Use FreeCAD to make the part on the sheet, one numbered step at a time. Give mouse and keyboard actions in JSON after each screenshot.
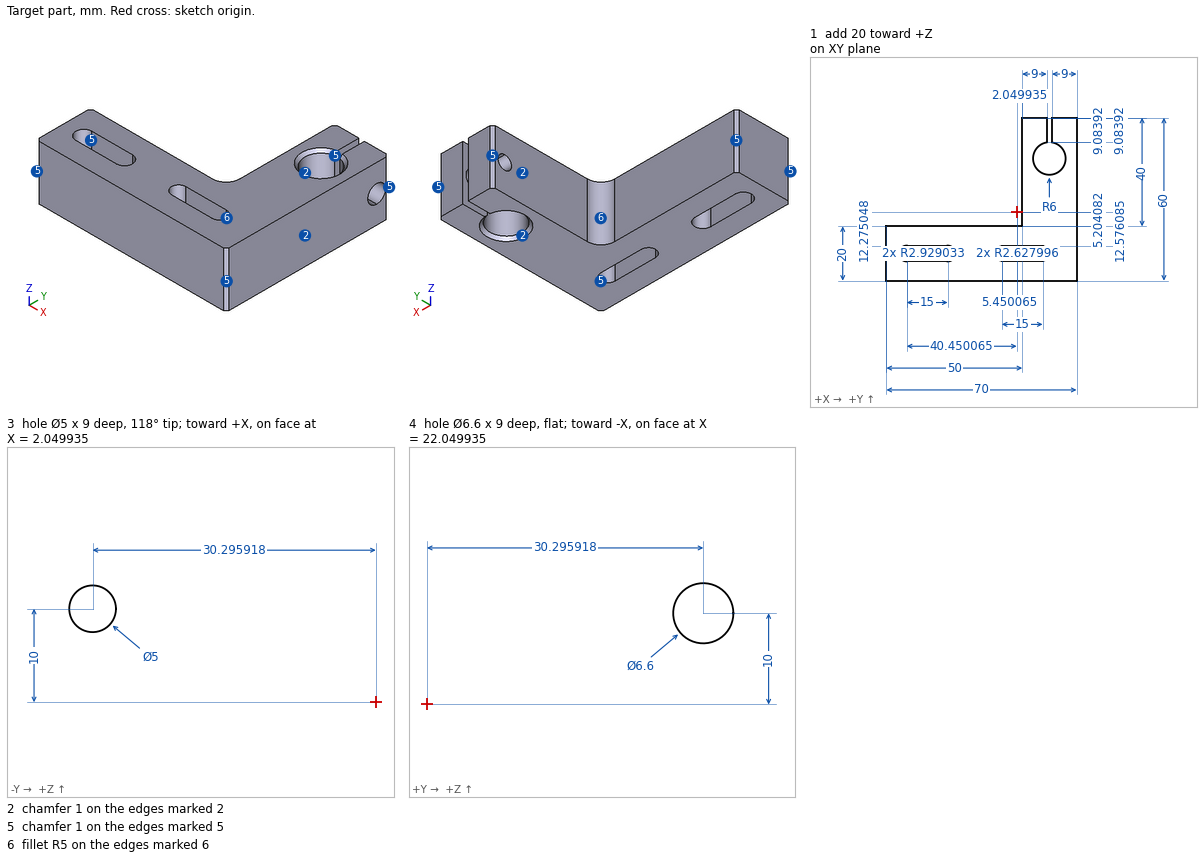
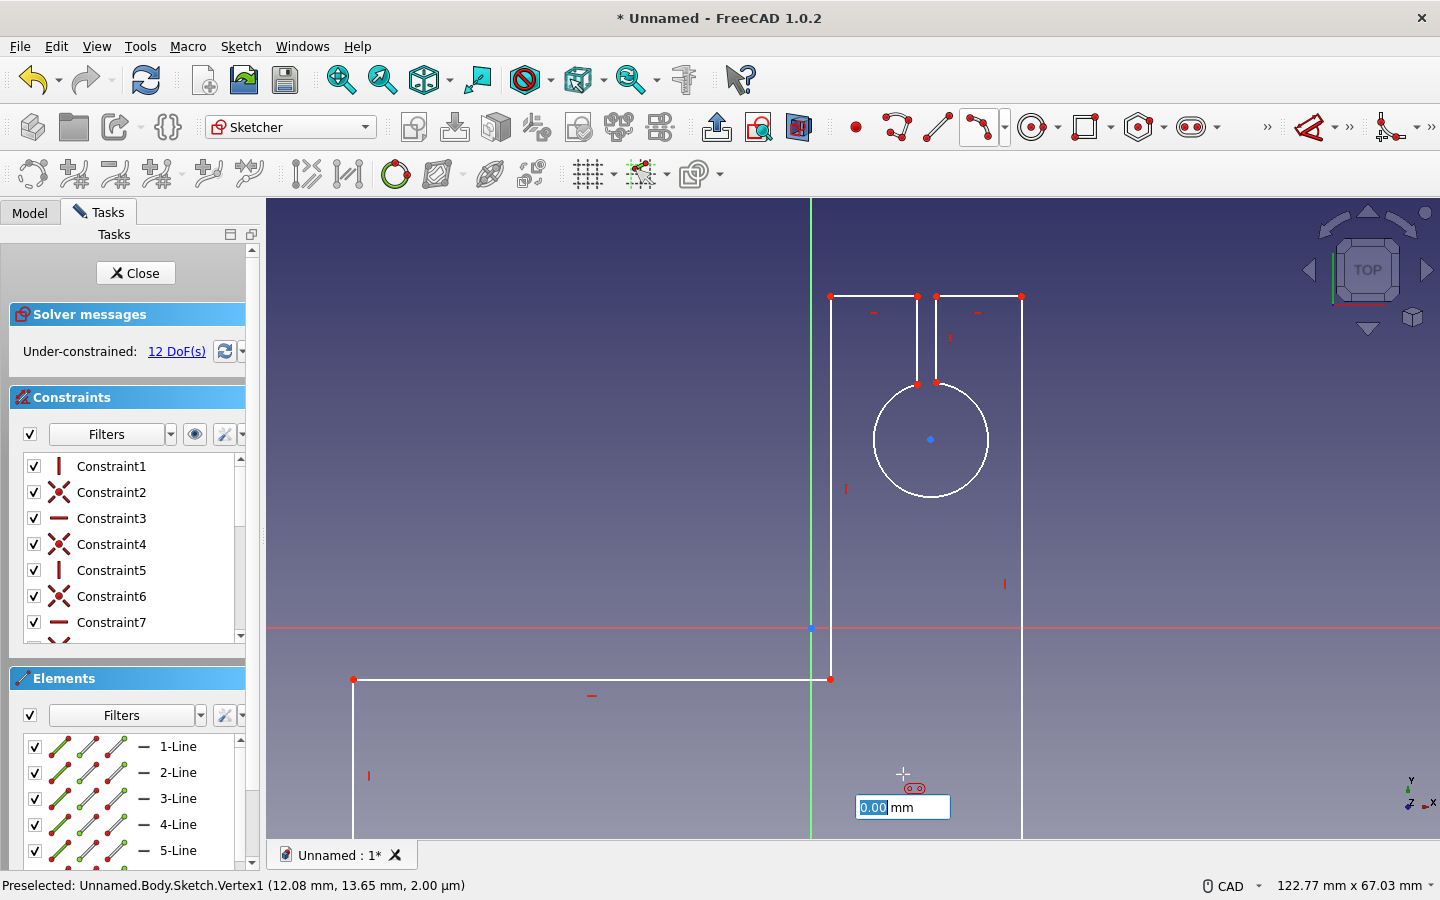
{"action": "left_click", "coordinate": [831, 749]}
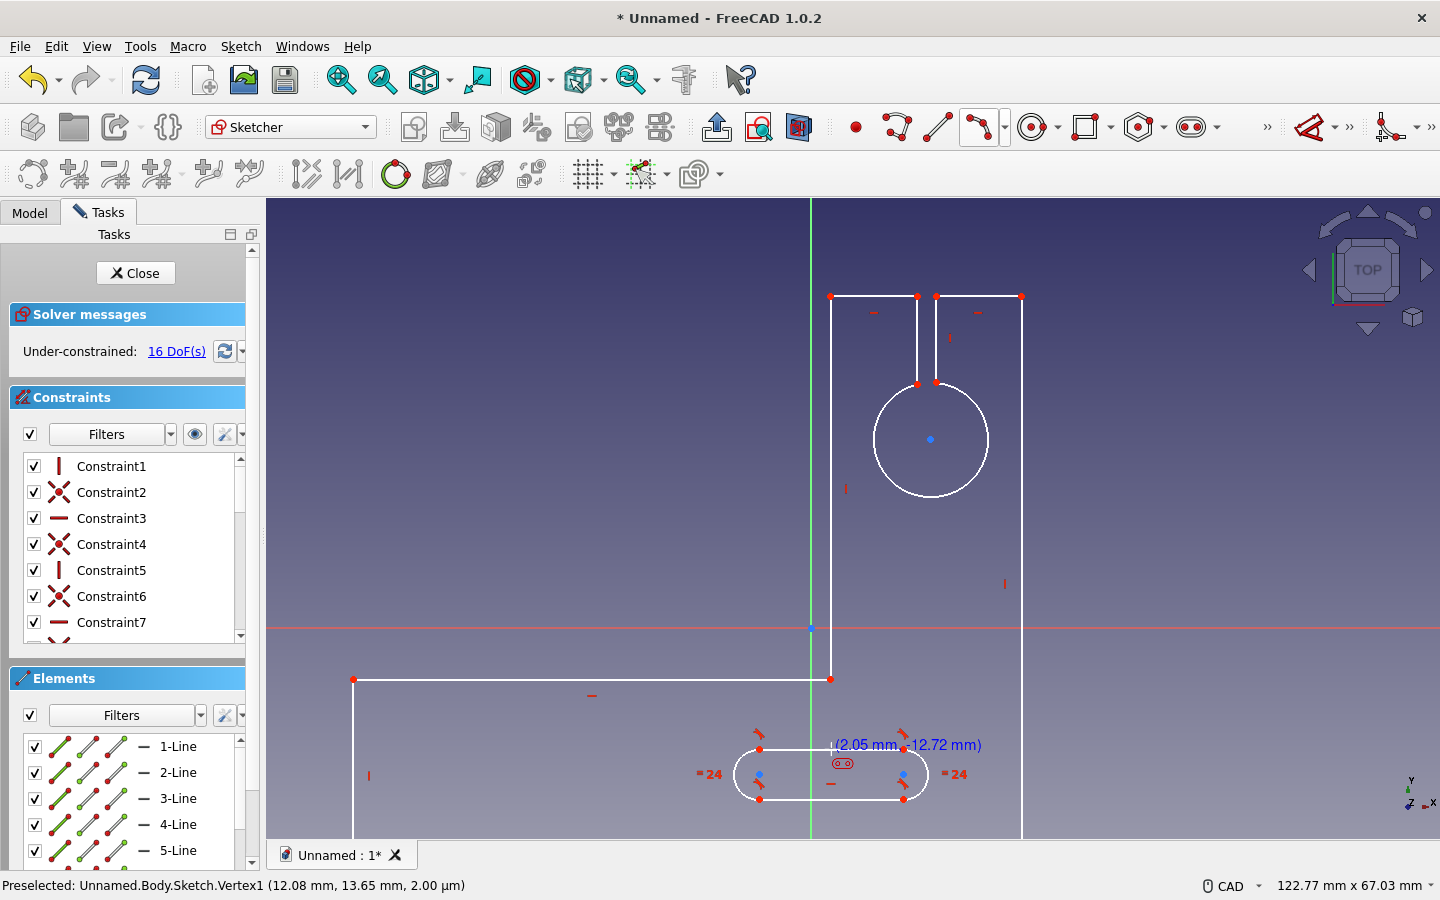
{"action": "left_click", "coordinate": [425, 774]}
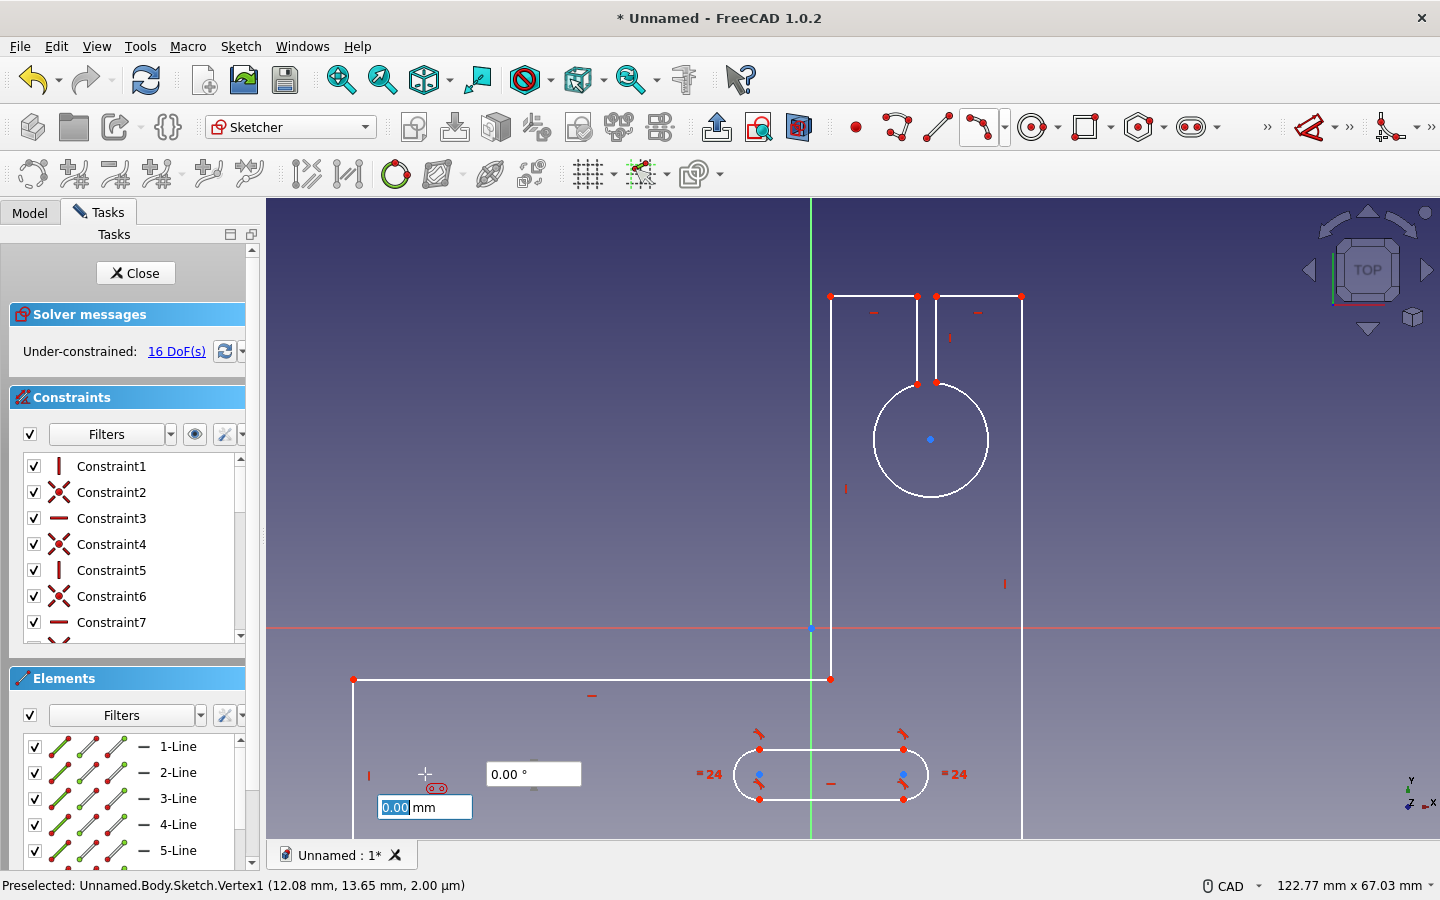
{"action": "left_click", "coordinate": [568, 774]}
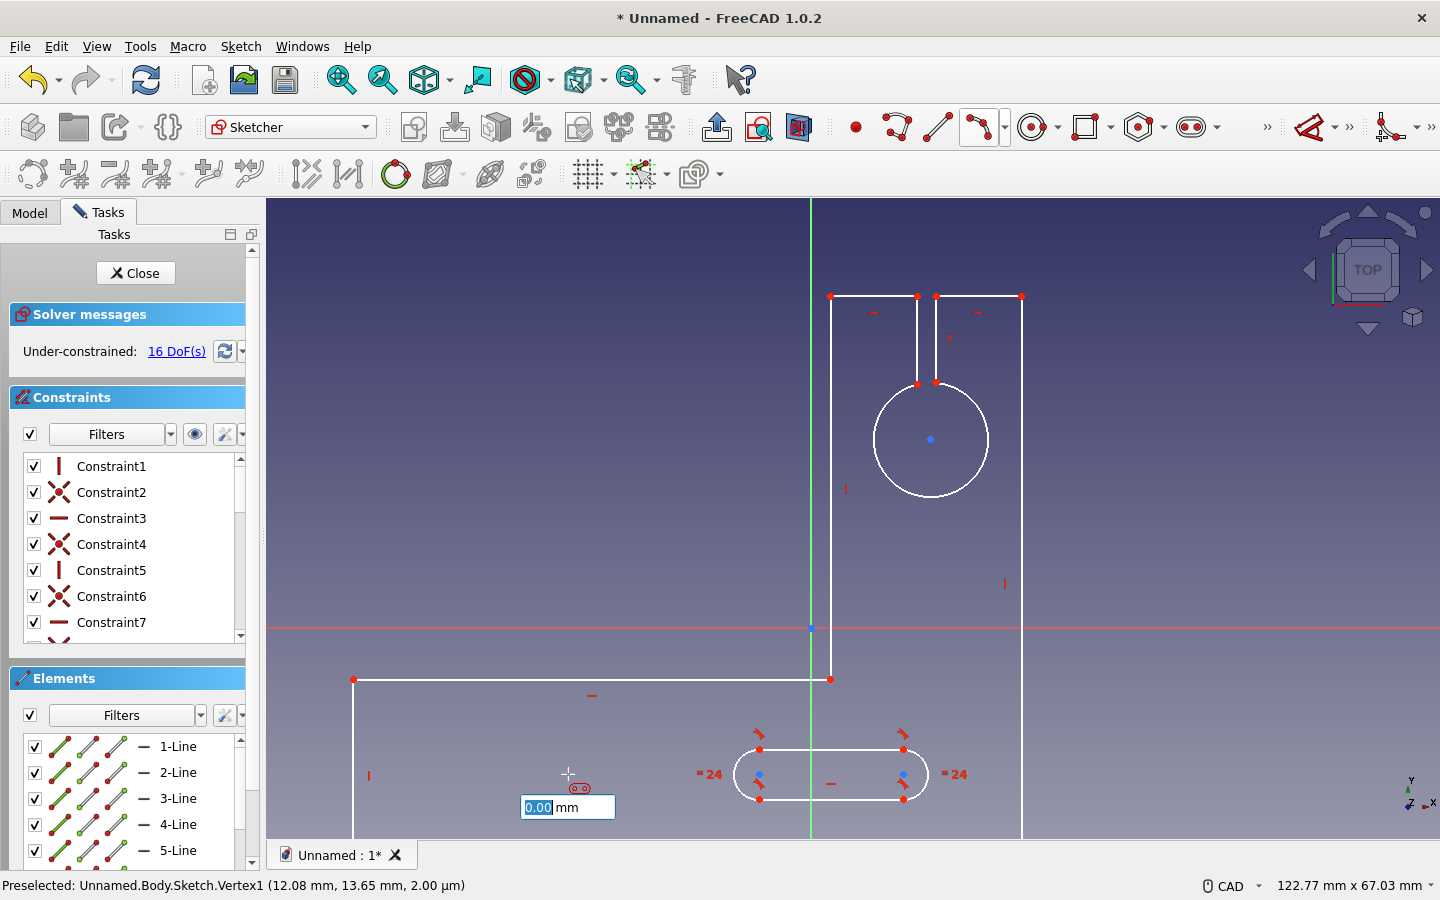
{"action": "left_click", "coordinate": [496, 746]}
{"action": "key", "text": "Escape"}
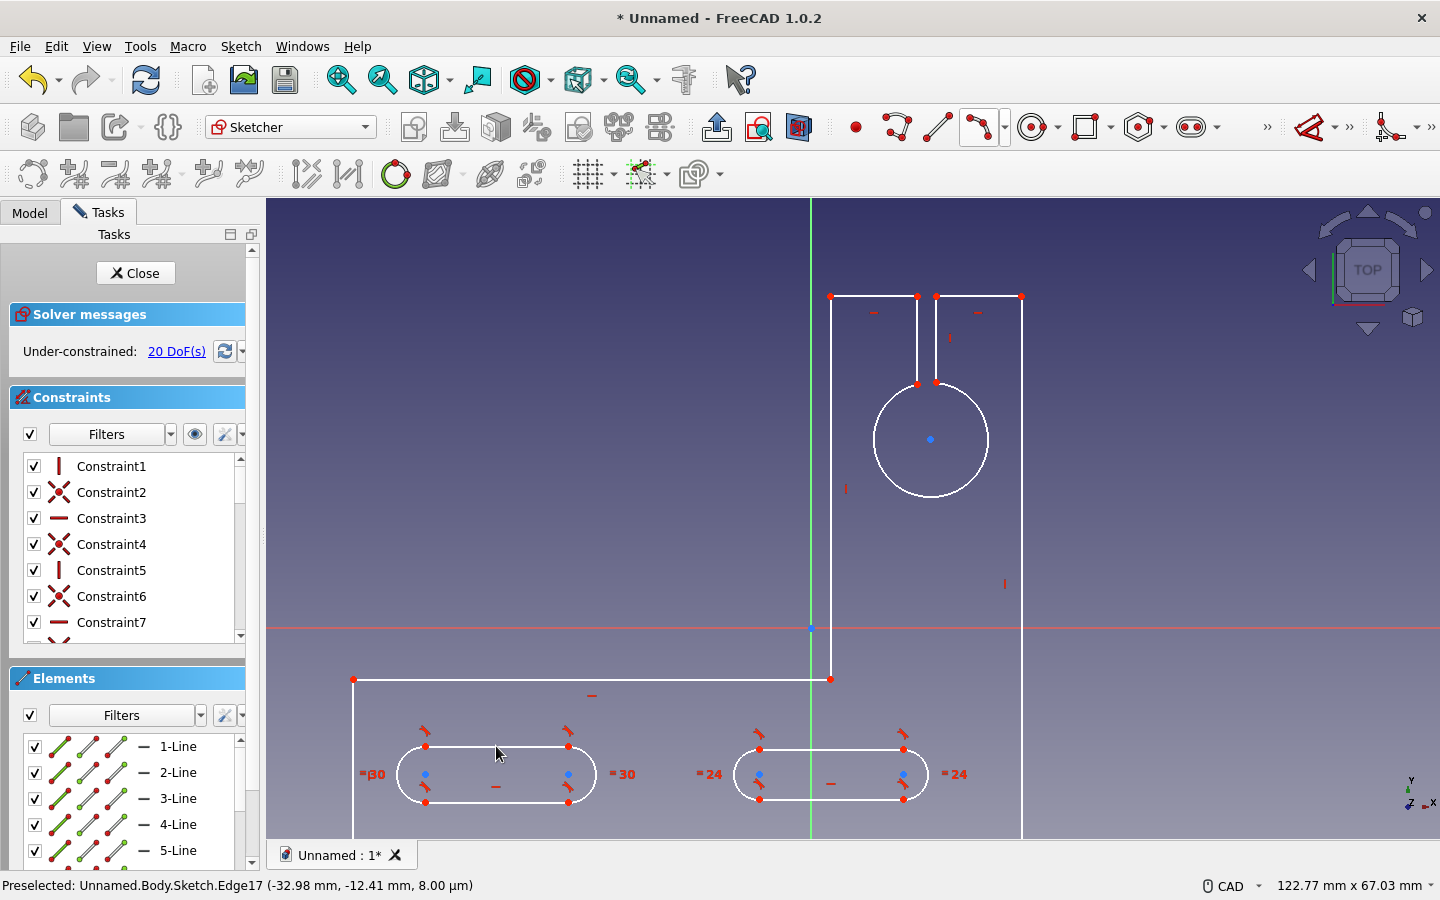
{"action": "left_click", "coordinate": [1308, 128]}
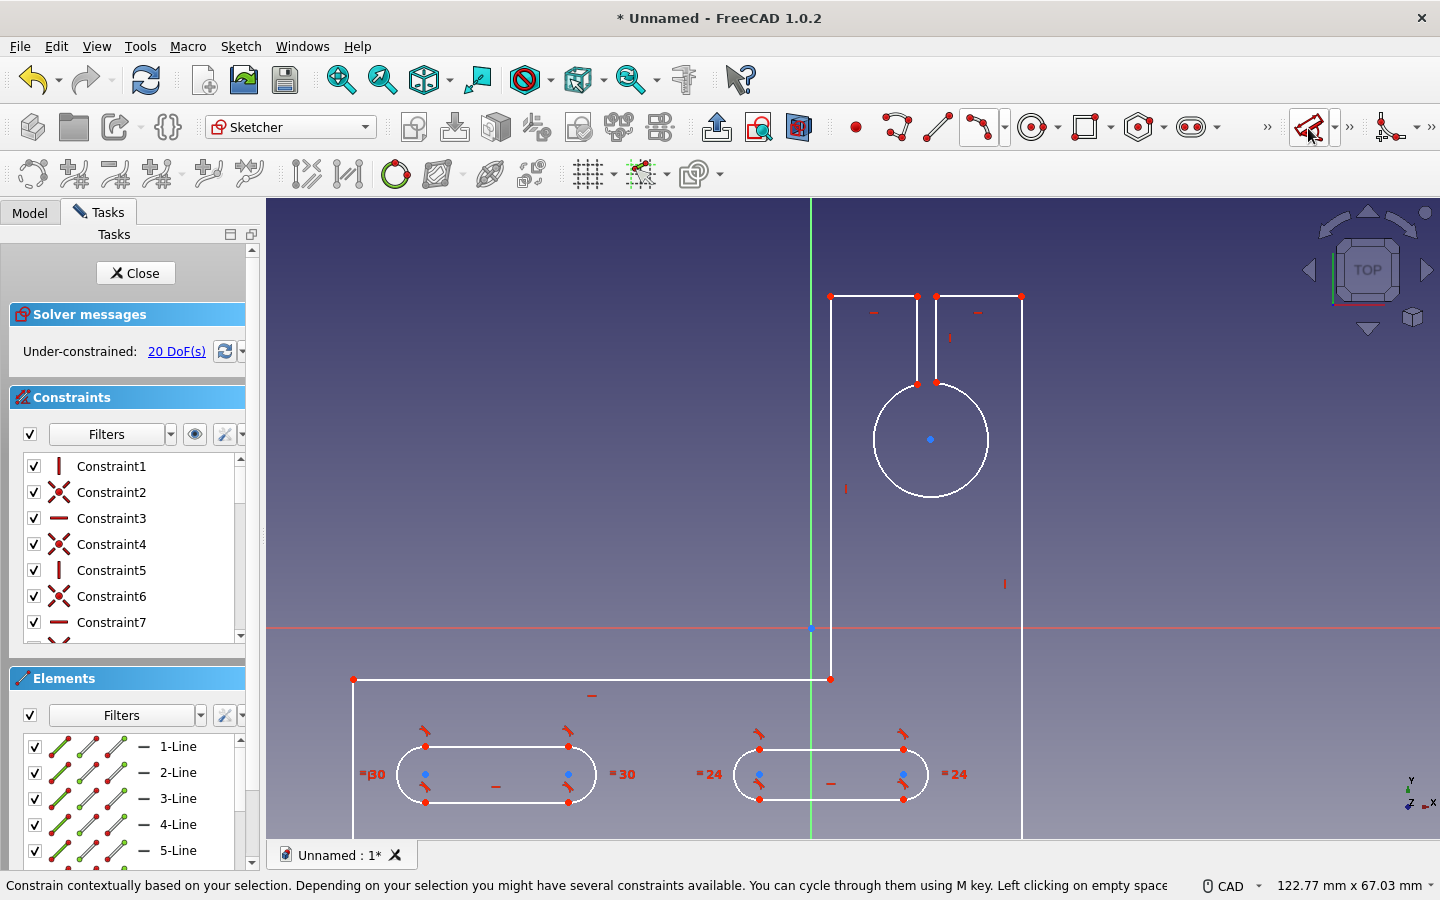
{"action": "left_click", "coordinate": [880, 465]}
{"action": "left_click", "coordinate": [851, 479]}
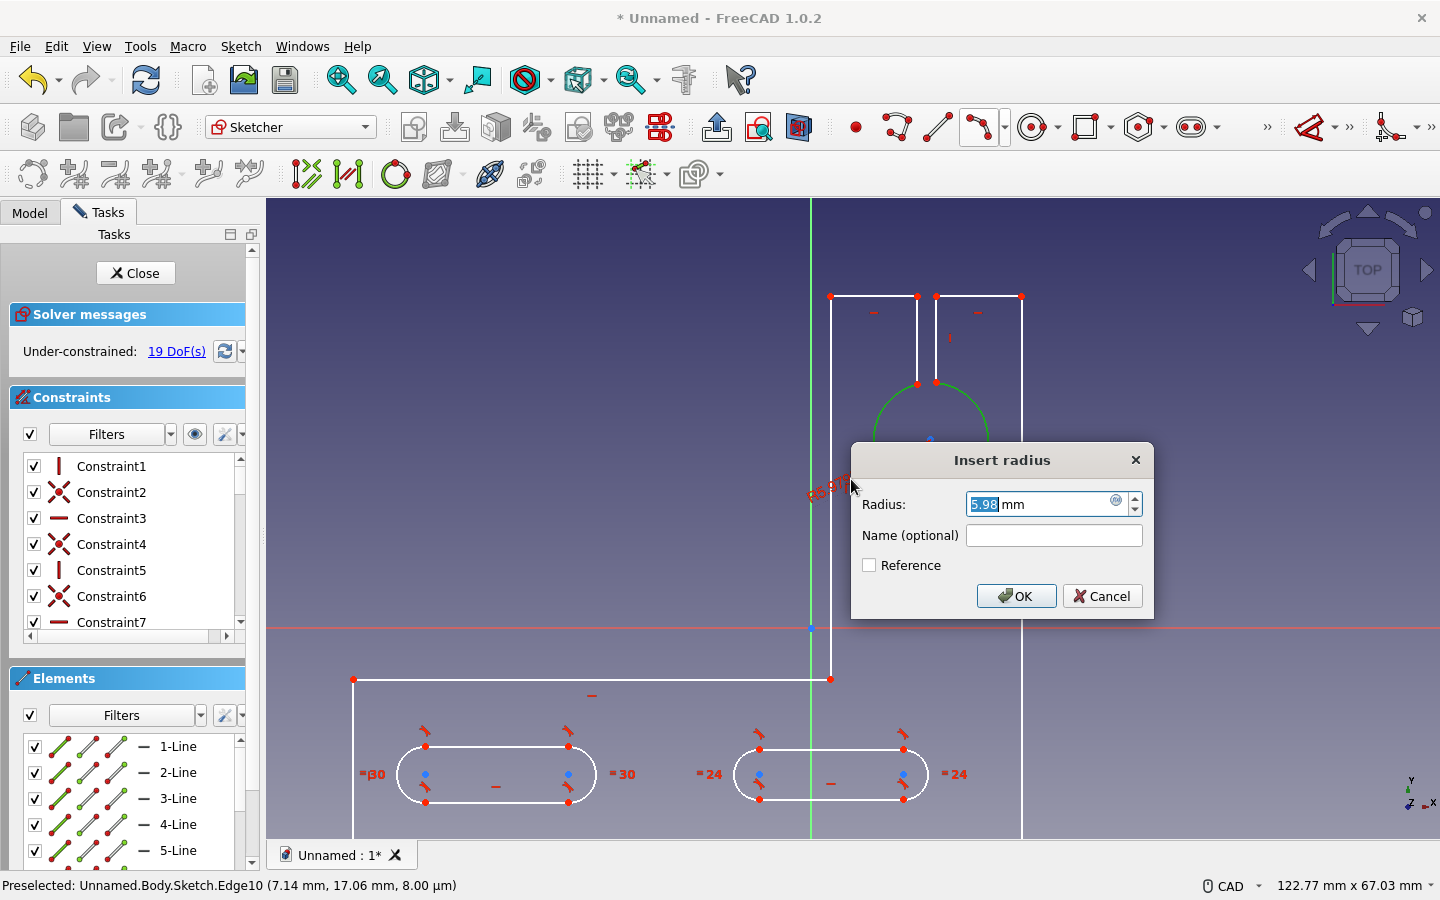
{"action": "type", "text": "6"}
{"action": "key", "text": "Return"}